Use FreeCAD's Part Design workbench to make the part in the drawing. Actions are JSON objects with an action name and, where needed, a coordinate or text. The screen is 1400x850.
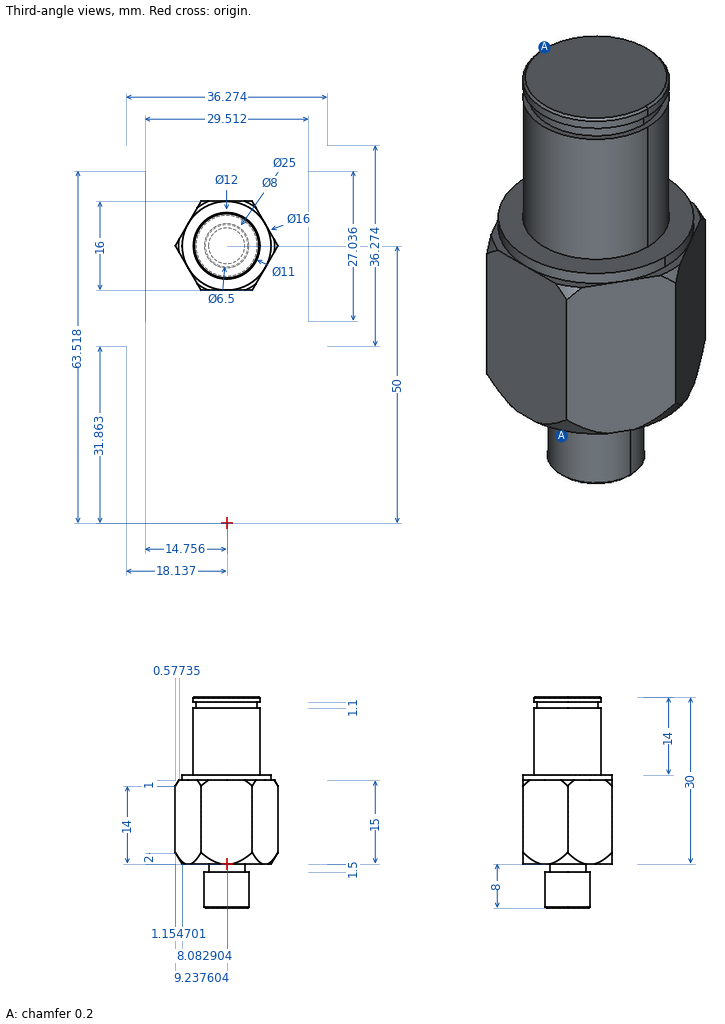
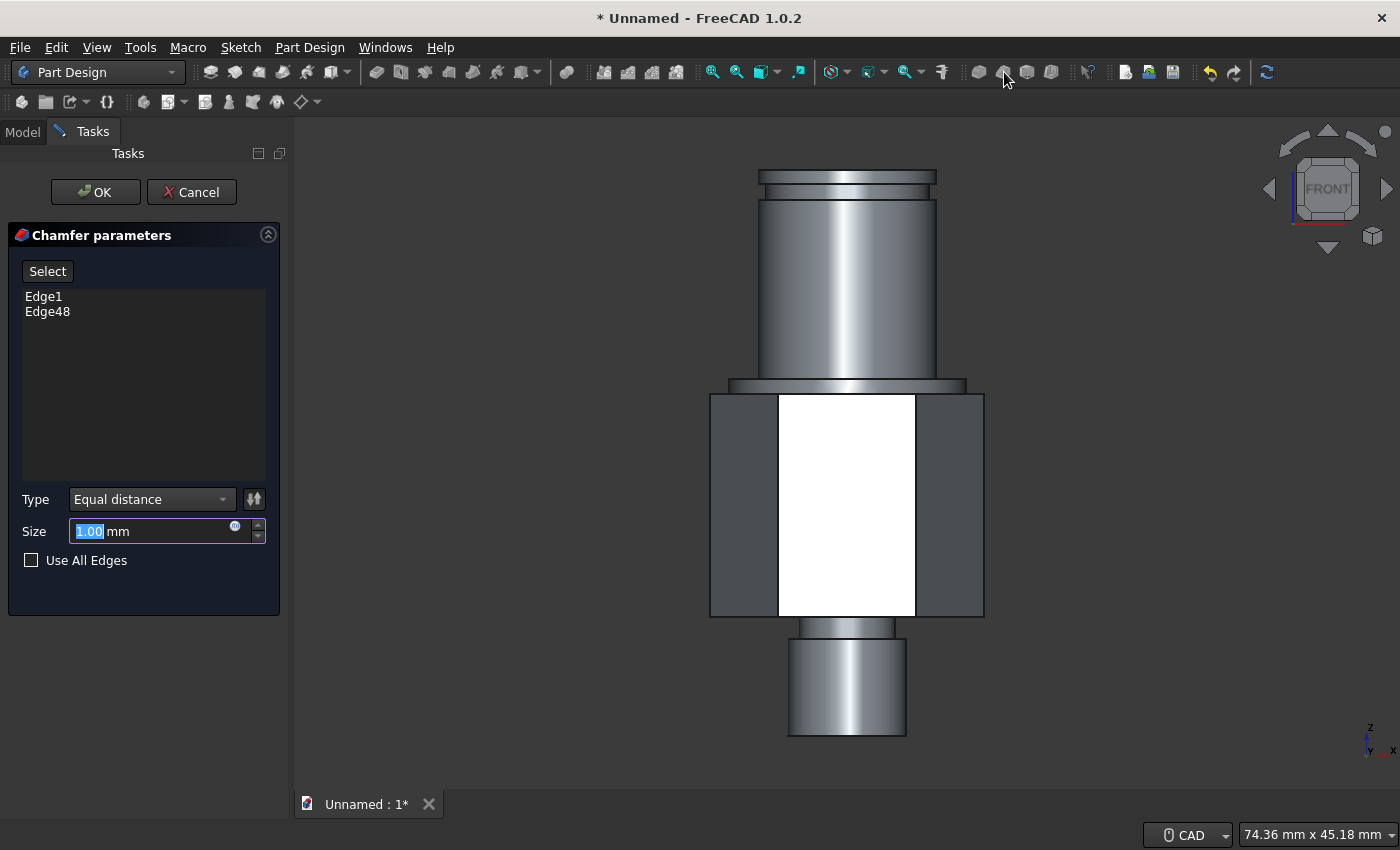
{"action": "type", "text": "0.2"}
{"action": "key", "text": "Tab"}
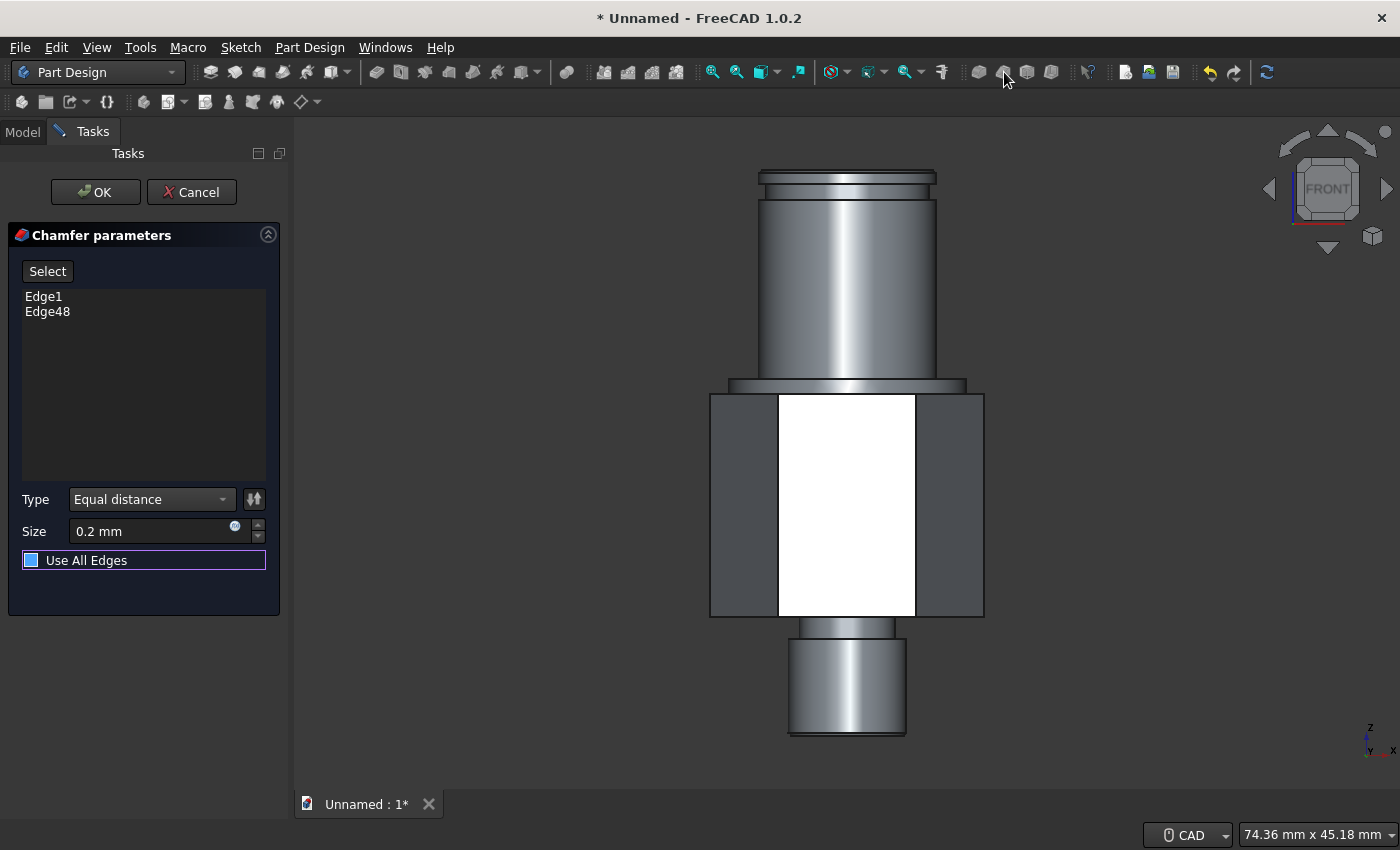
{"action": "left_click", "coordinate": [96, 192]}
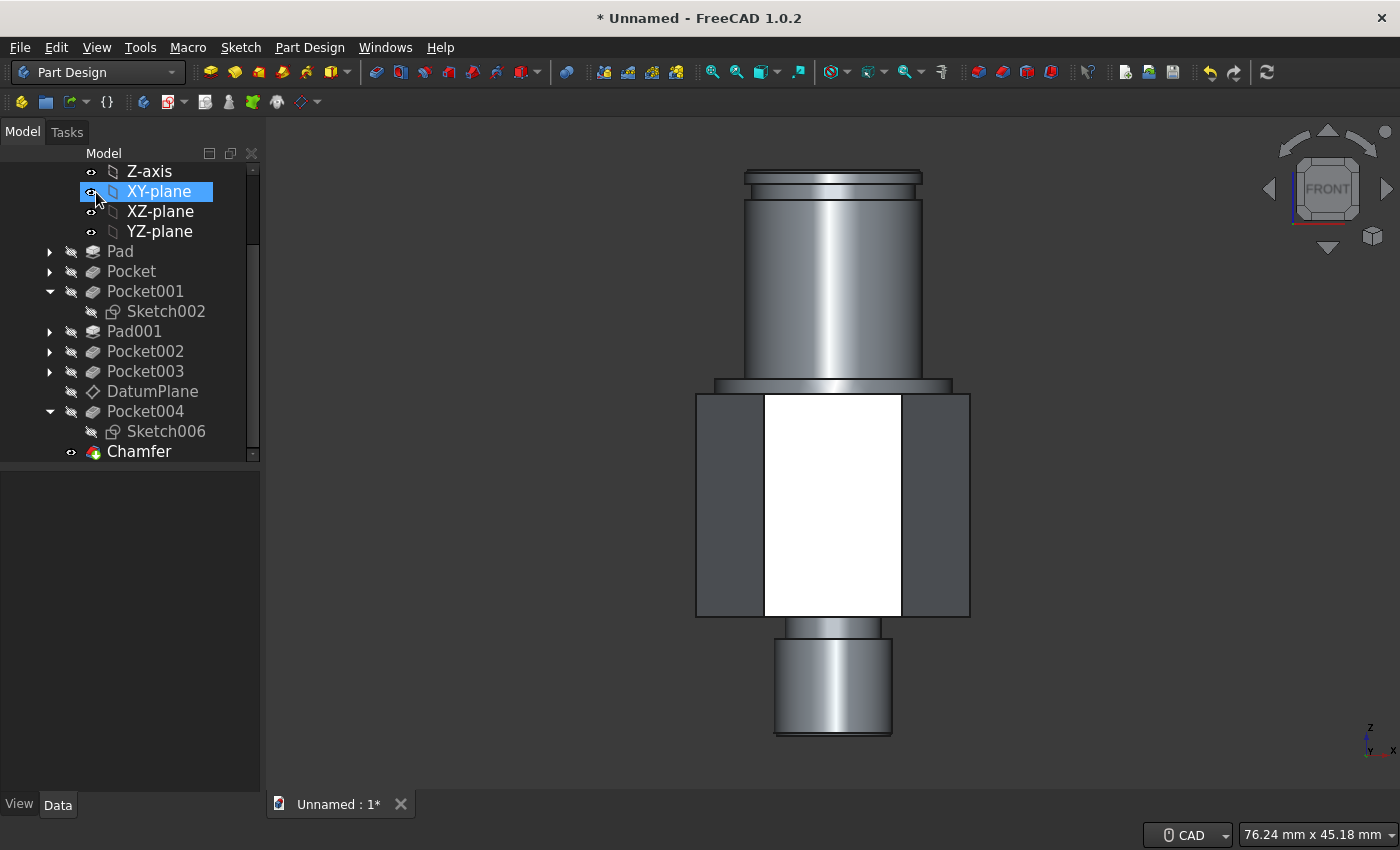
{"action": "scroll", "coordinate": [160, 307], "scroll_direction": "down", "scroll_amount": 3}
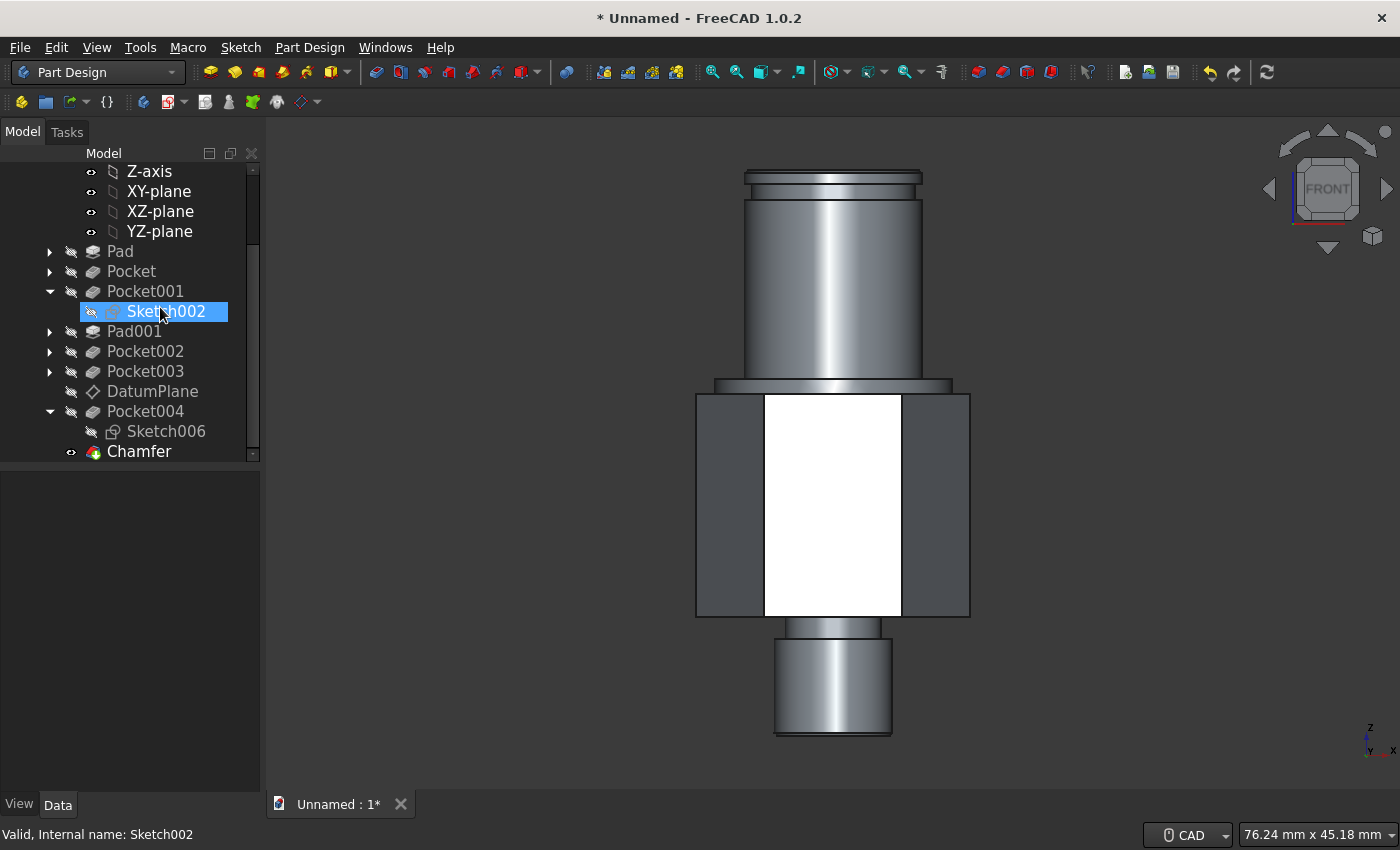
{"action": "scroll", "coordinate": [160, 307], "scroll_direction": "up", "scroll_amount": 15}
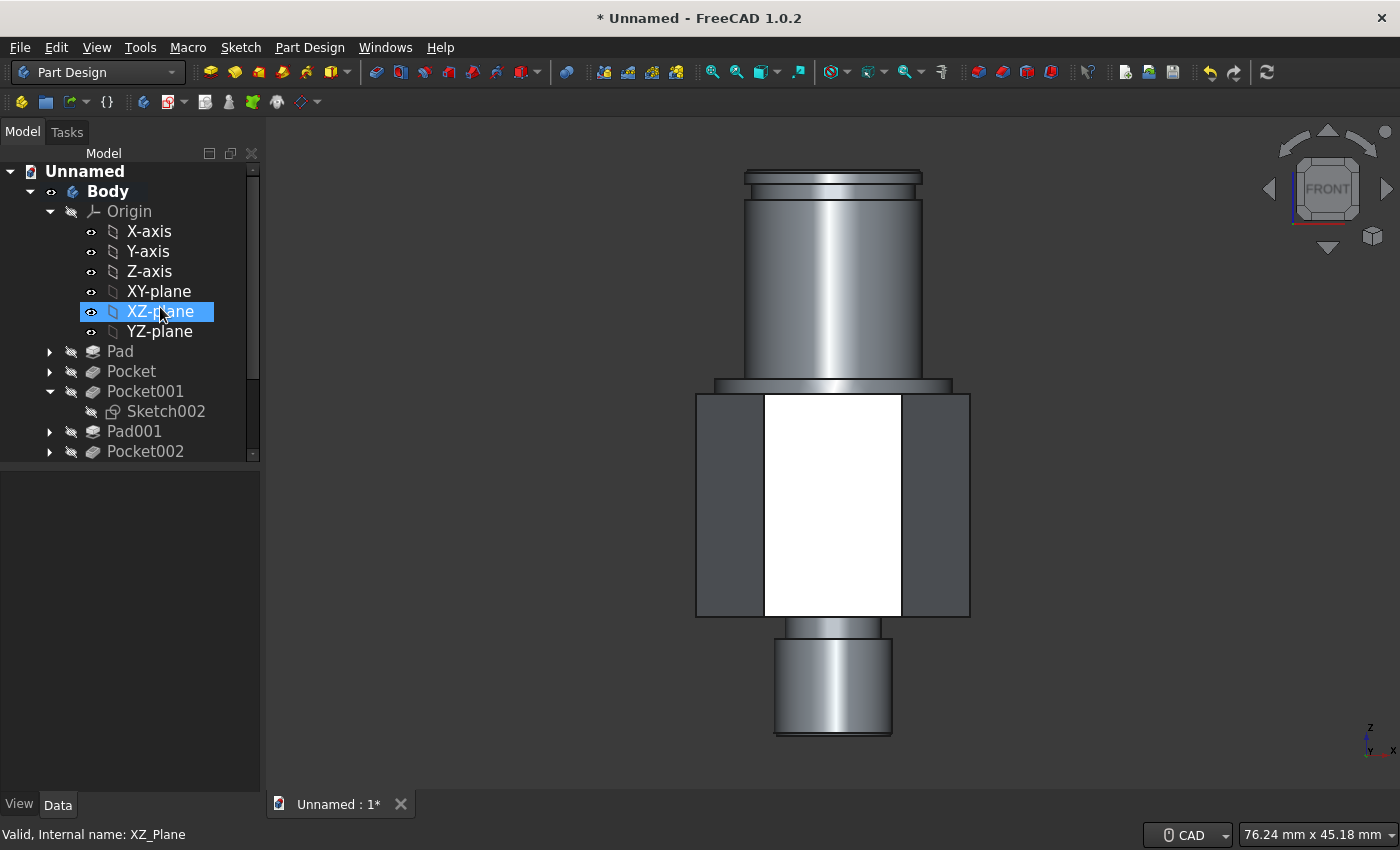
{"action": "left_click", "coordinate": [136, 312]}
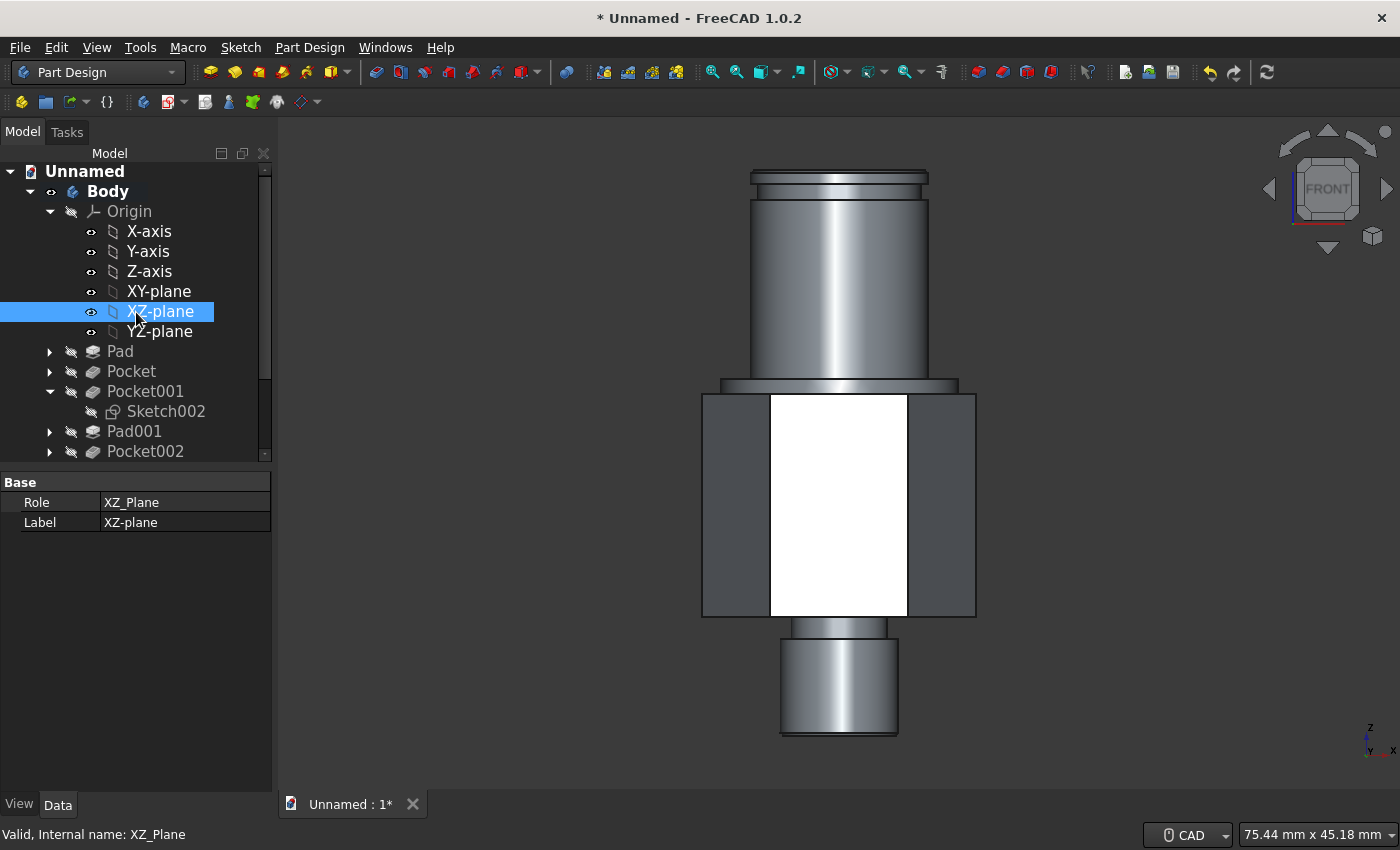
{"action": "left_click", "coordinate": [302, 102]}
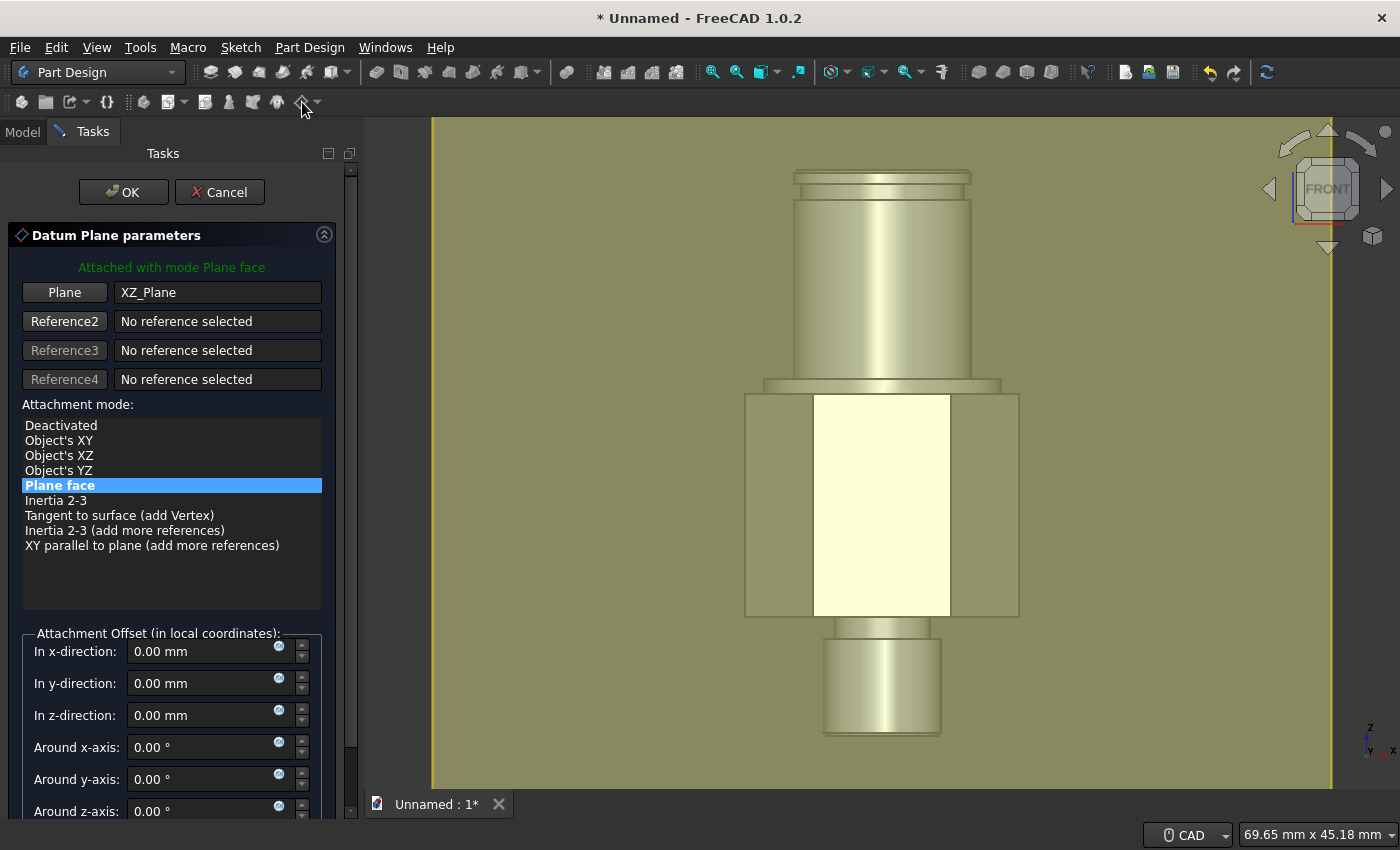
{"action": "triple_click", "coordinate": [210, 715]}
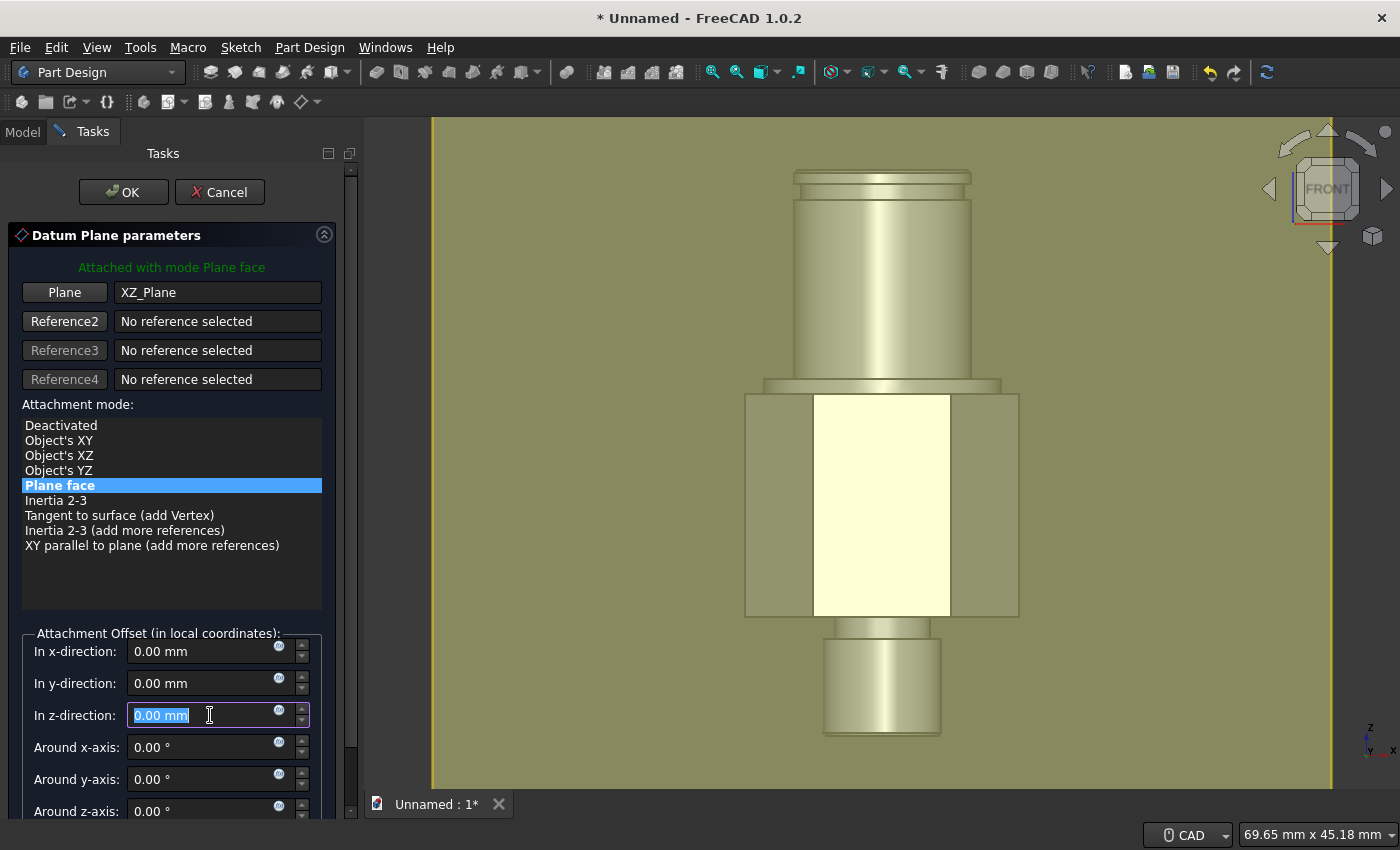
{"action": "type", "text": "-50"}
{"action": "key", "text": "Tab"}